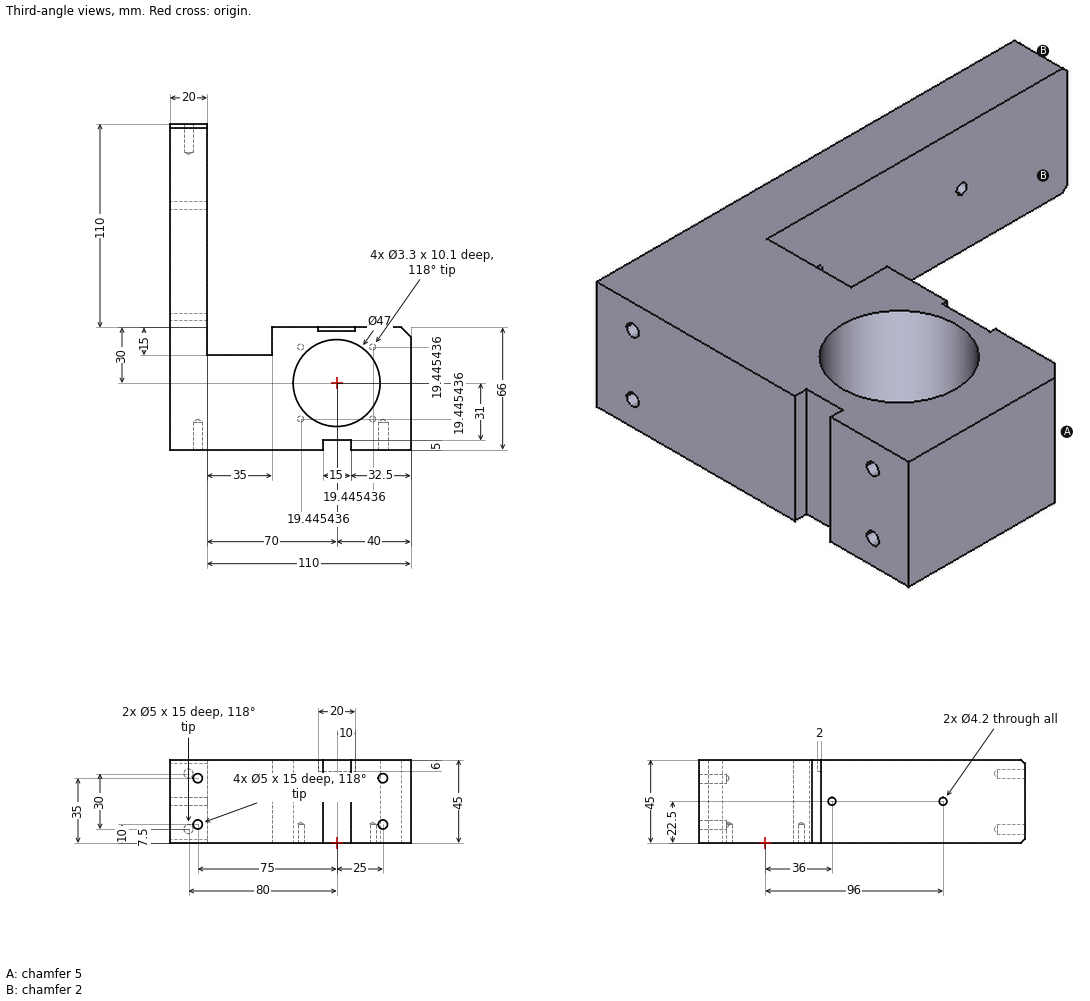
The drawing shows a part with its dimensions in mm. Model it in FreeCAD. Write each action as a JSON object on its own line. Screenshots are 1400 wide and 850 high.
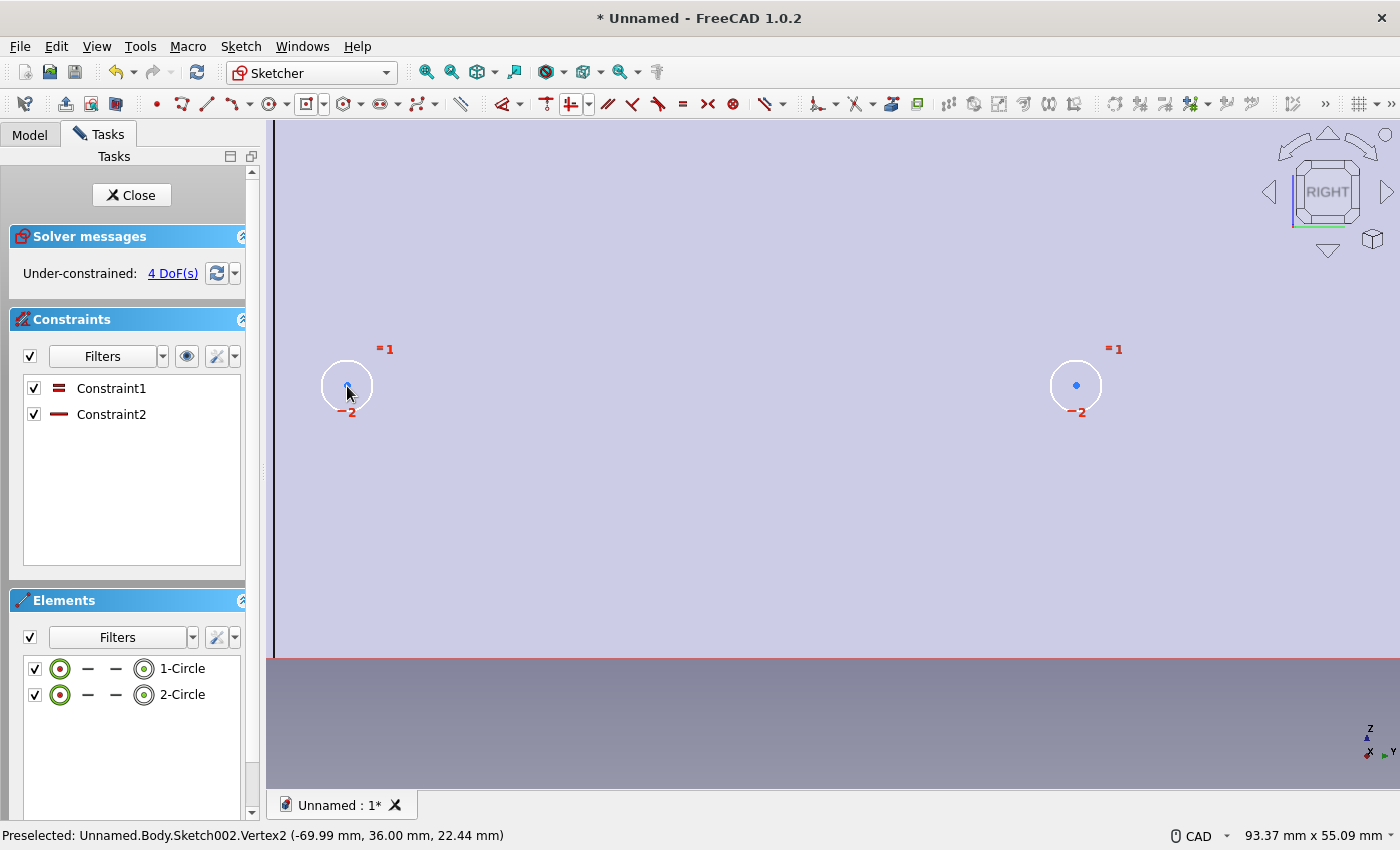
{"action": "left_click", "coordinate": [502, 104]}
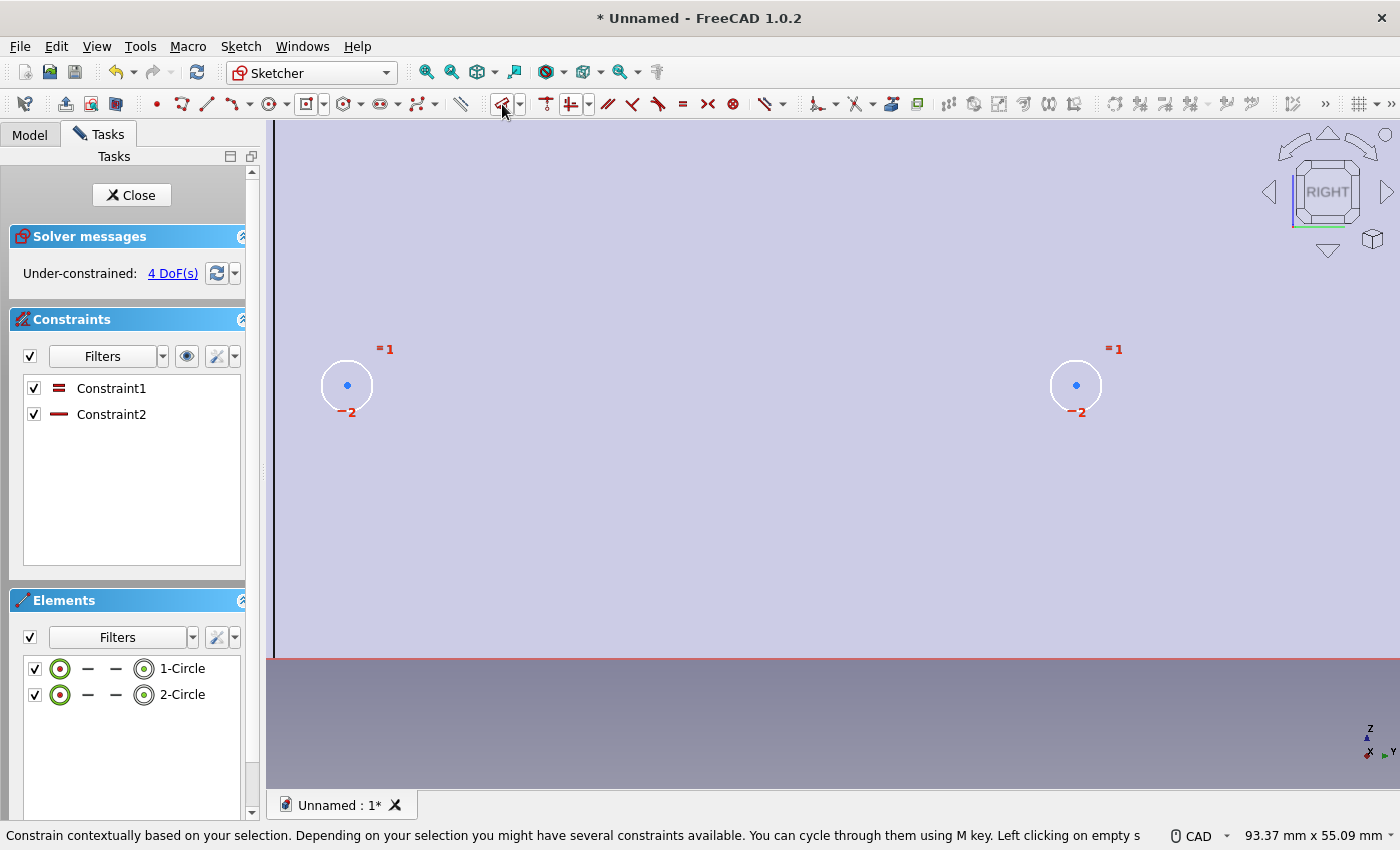
{"action": "left_click", "coordinate": [1094, 368]}
{"action": "left_click", "coordinate": [1117, 345]}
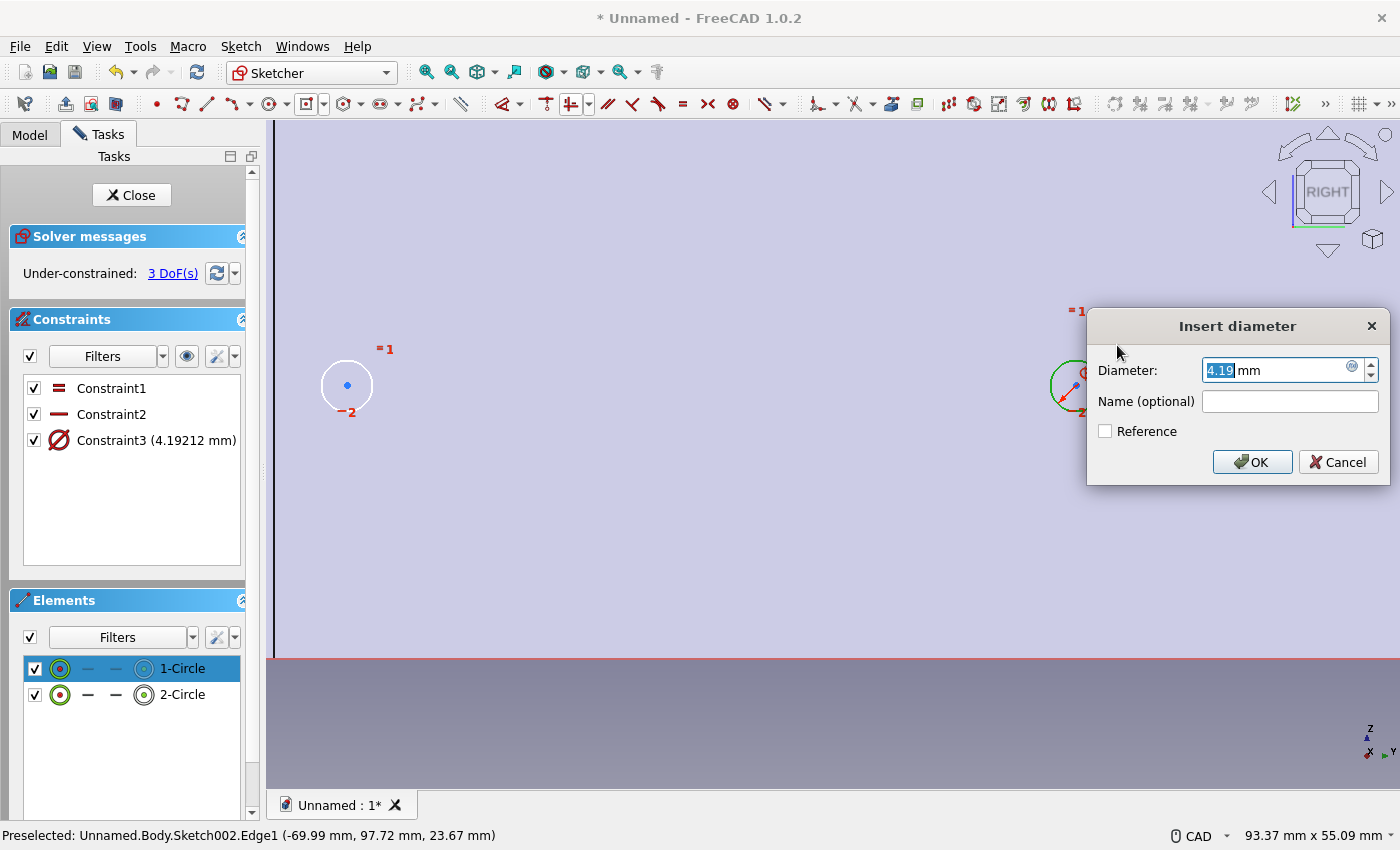
{"action": "type", "text": "4.2"}
{"action": "key", "text": "Return"}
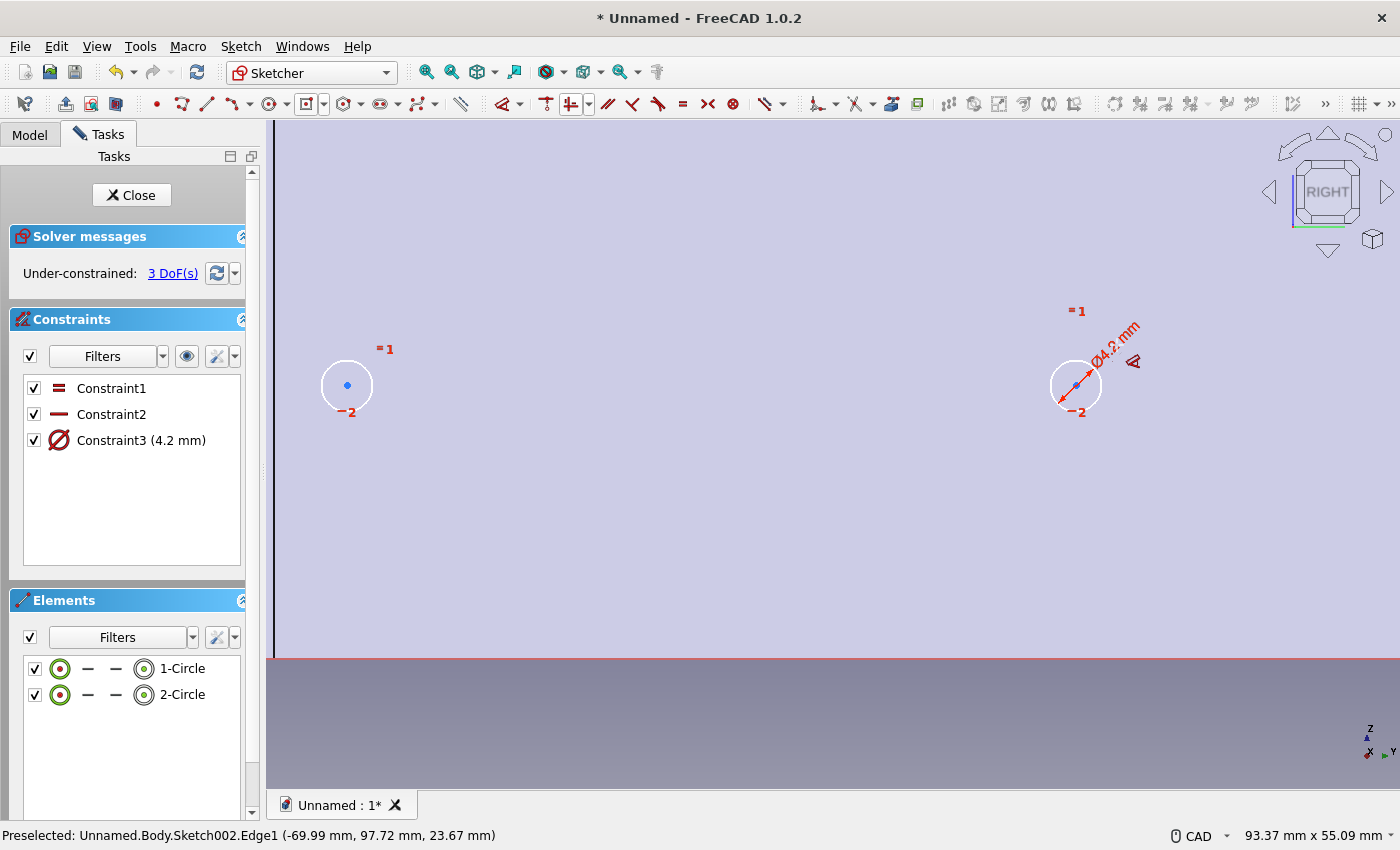
{"action": "left_click", "coordinate": [1076, 386]}
{"action": "left_click", "coordinate": [685, 693]}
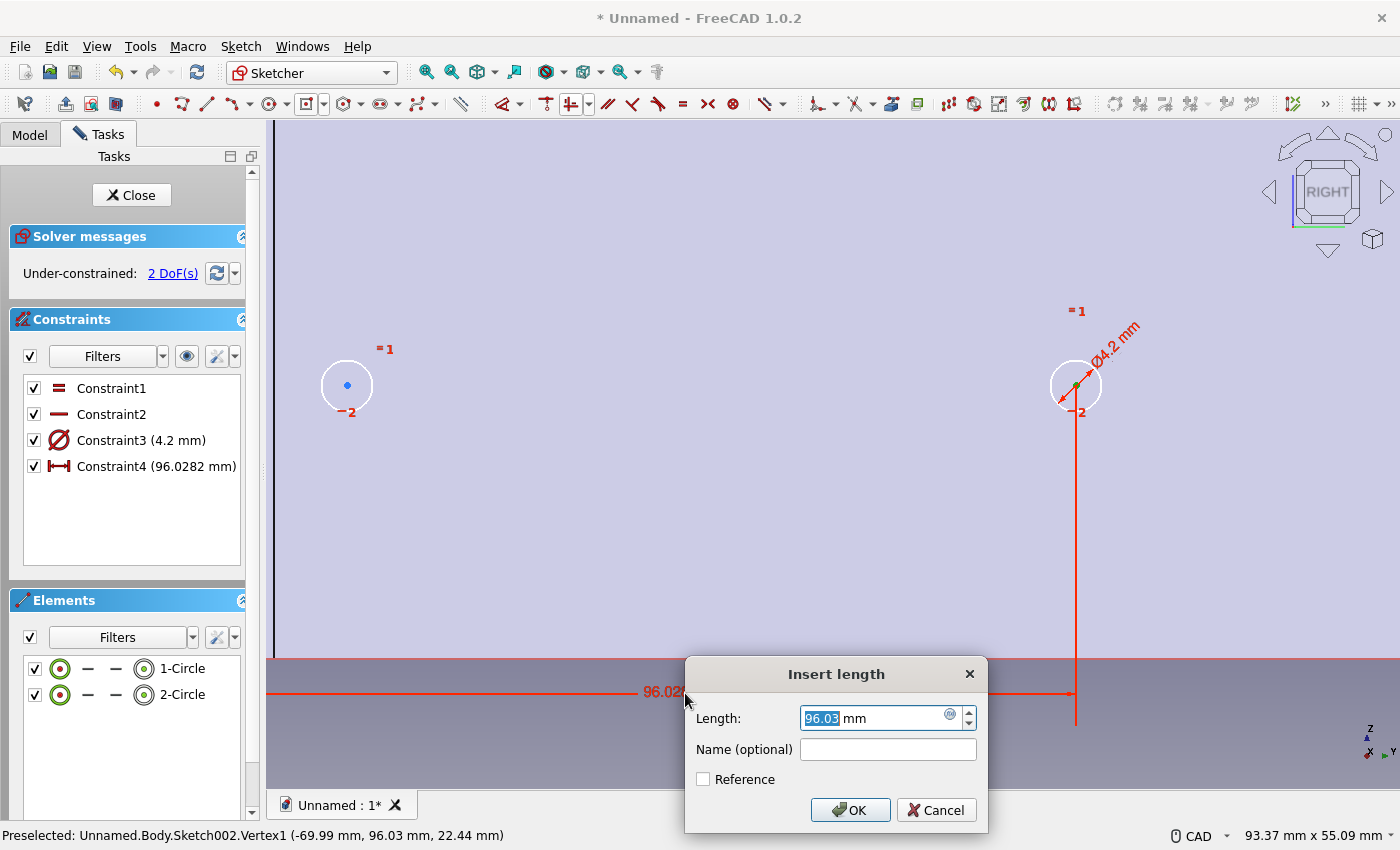
{"action": "type", "text": "96"}
{"action": "key", "text": "Return"}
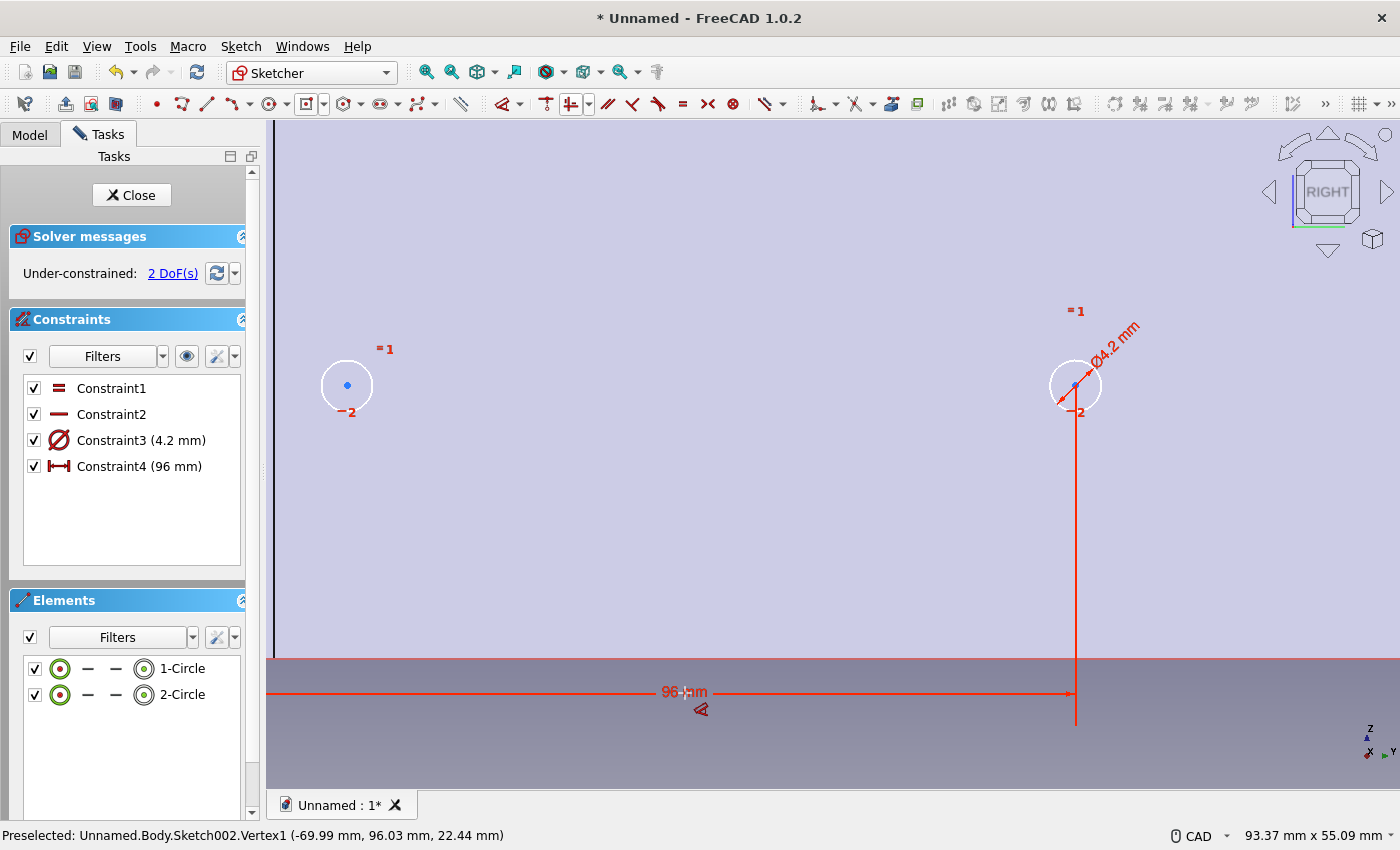
{"action": "left_click", "coordinate": [347, 386]}
{"action": "left_click", "coordinate": [320, 693]}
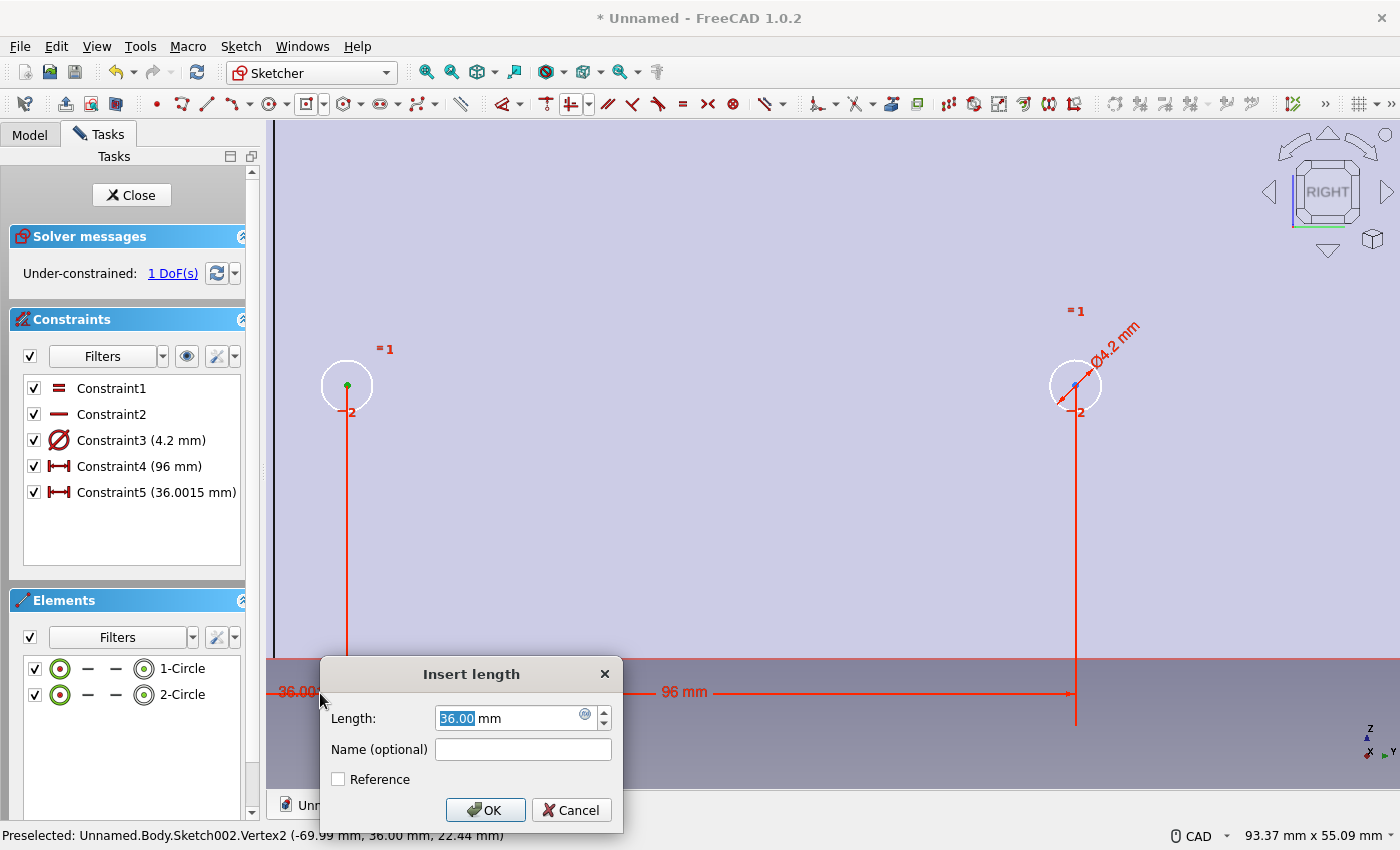
{"action": "type", "text": "36"}
{"action": "key", "text": "Return"}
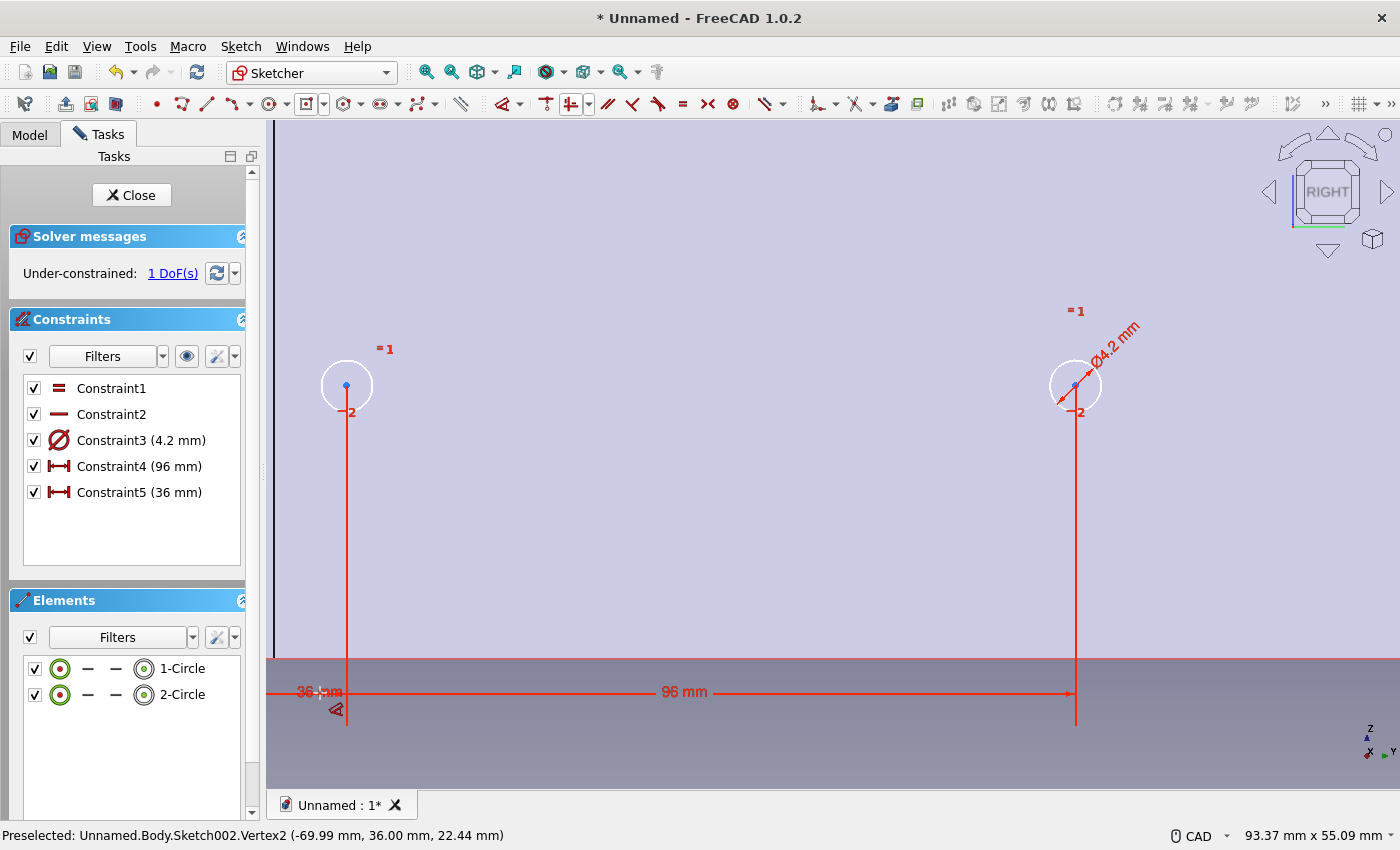
{"action": "left_click", "coordinate": [1076, 386]}
{"action": "left_click", "coordinate": [1110, 522]}